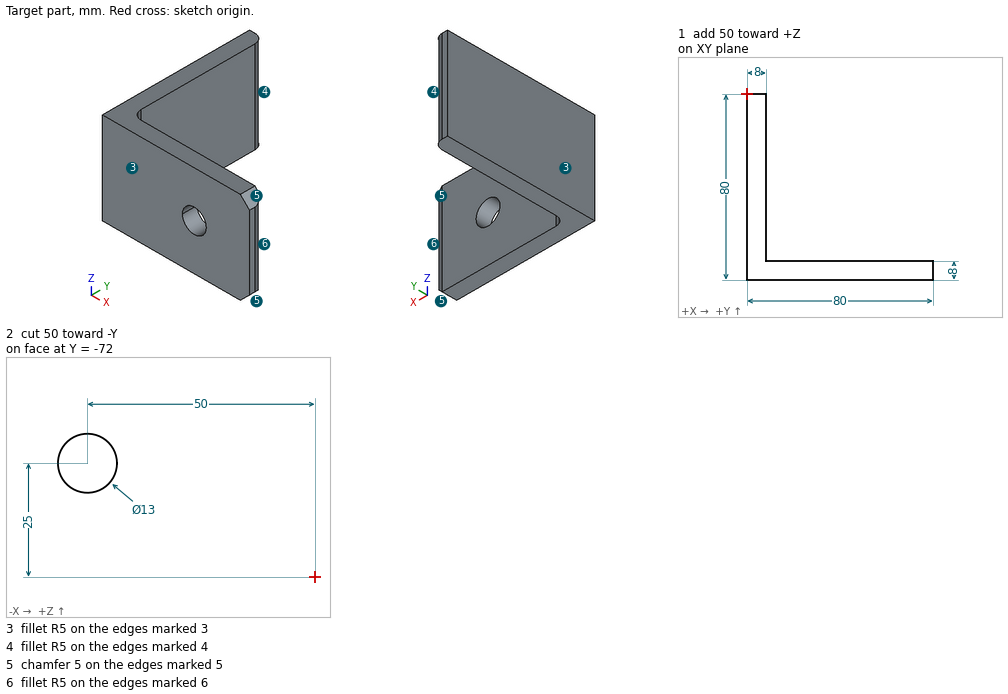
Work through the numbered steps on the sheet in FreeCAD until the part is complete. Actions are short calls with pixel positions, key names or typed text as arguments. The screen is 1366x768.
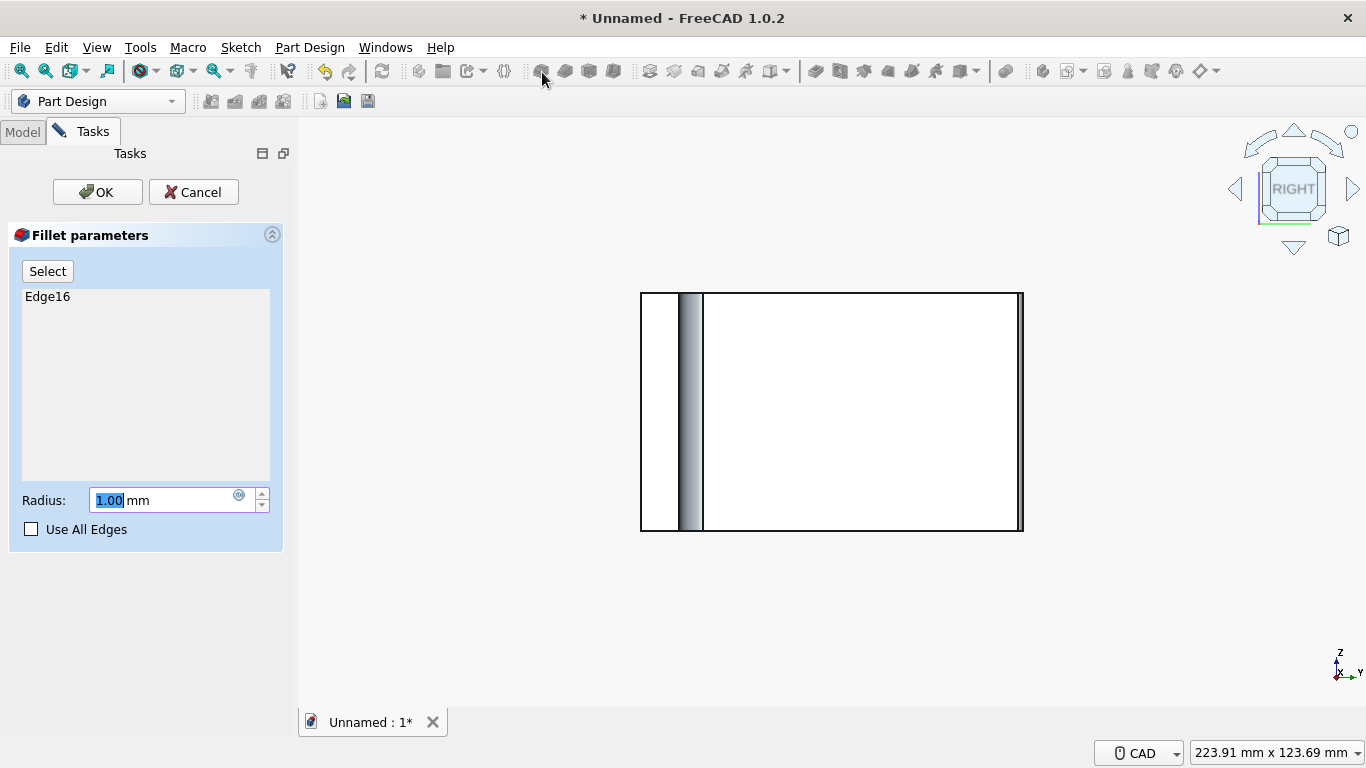
text(5)
key(Tab)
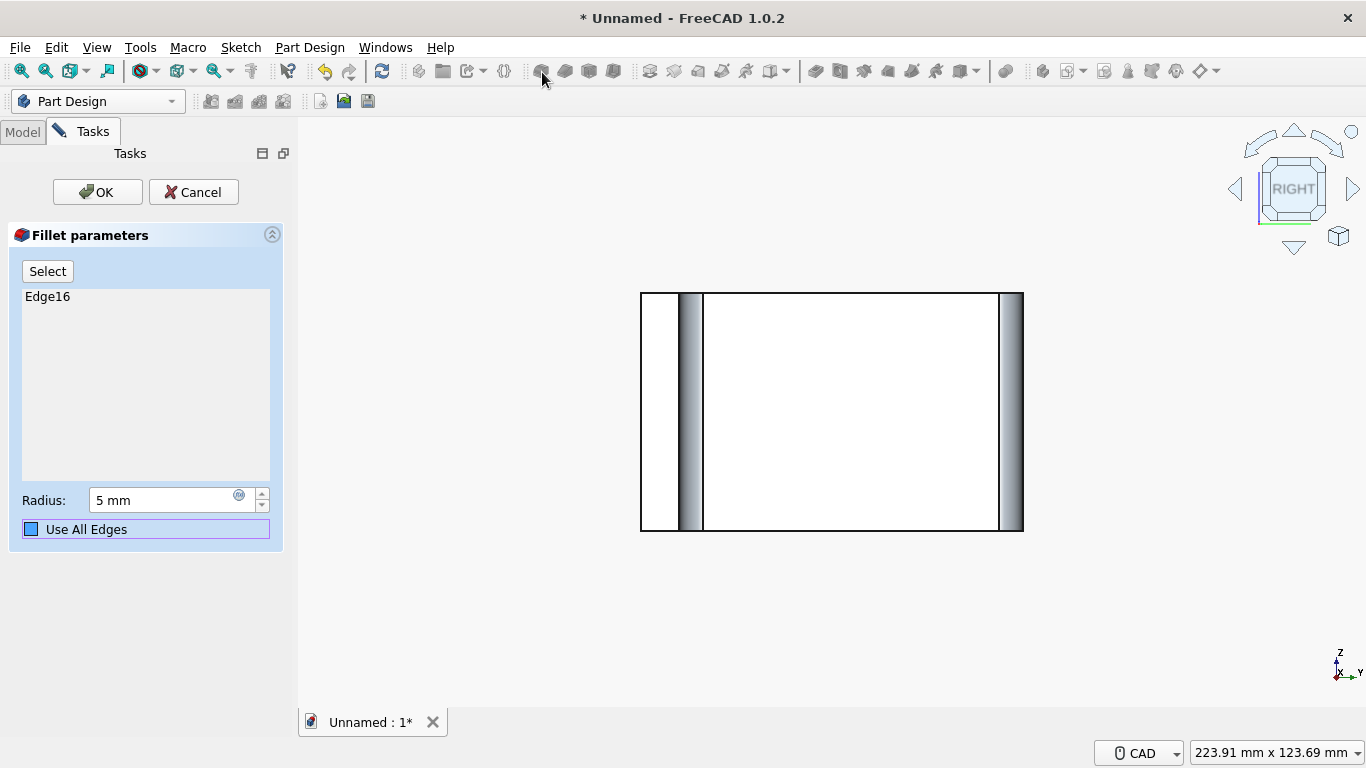
click(98, 192)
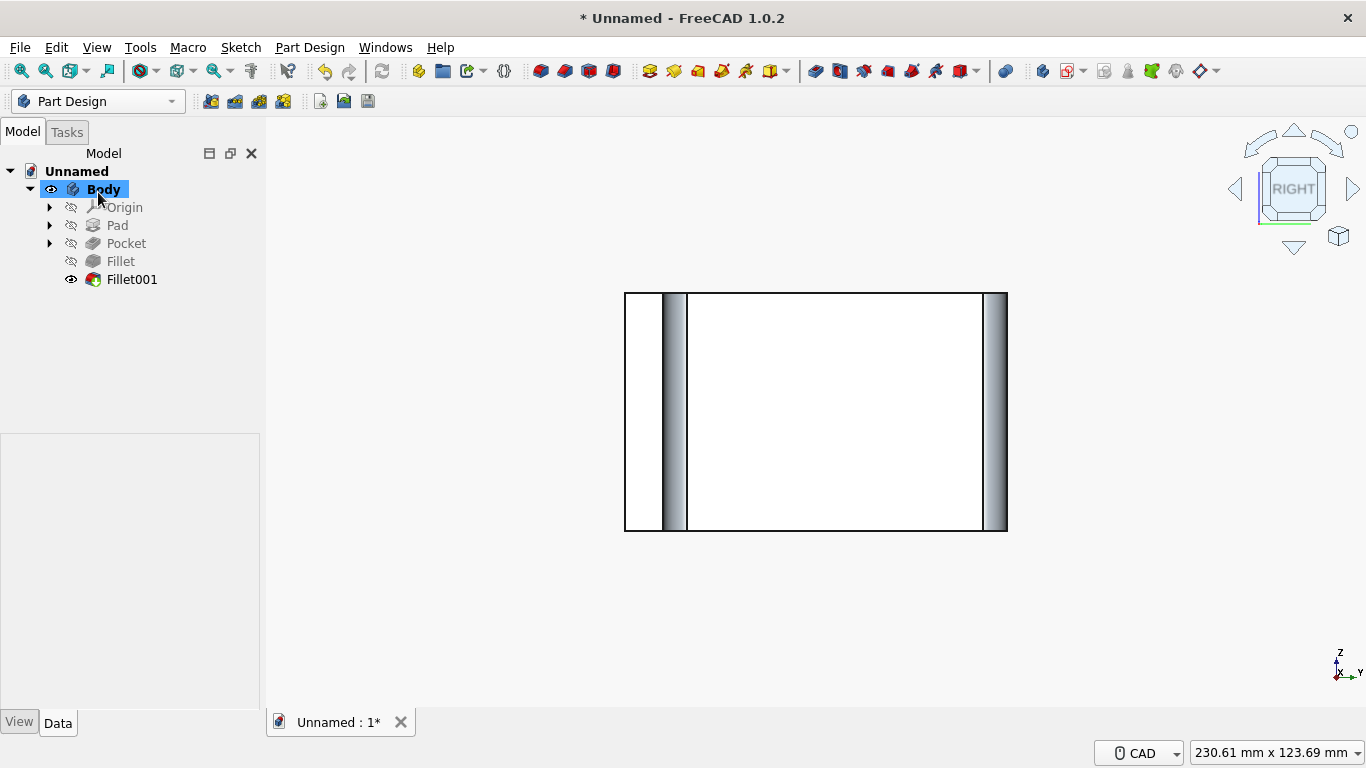
click(22, 72)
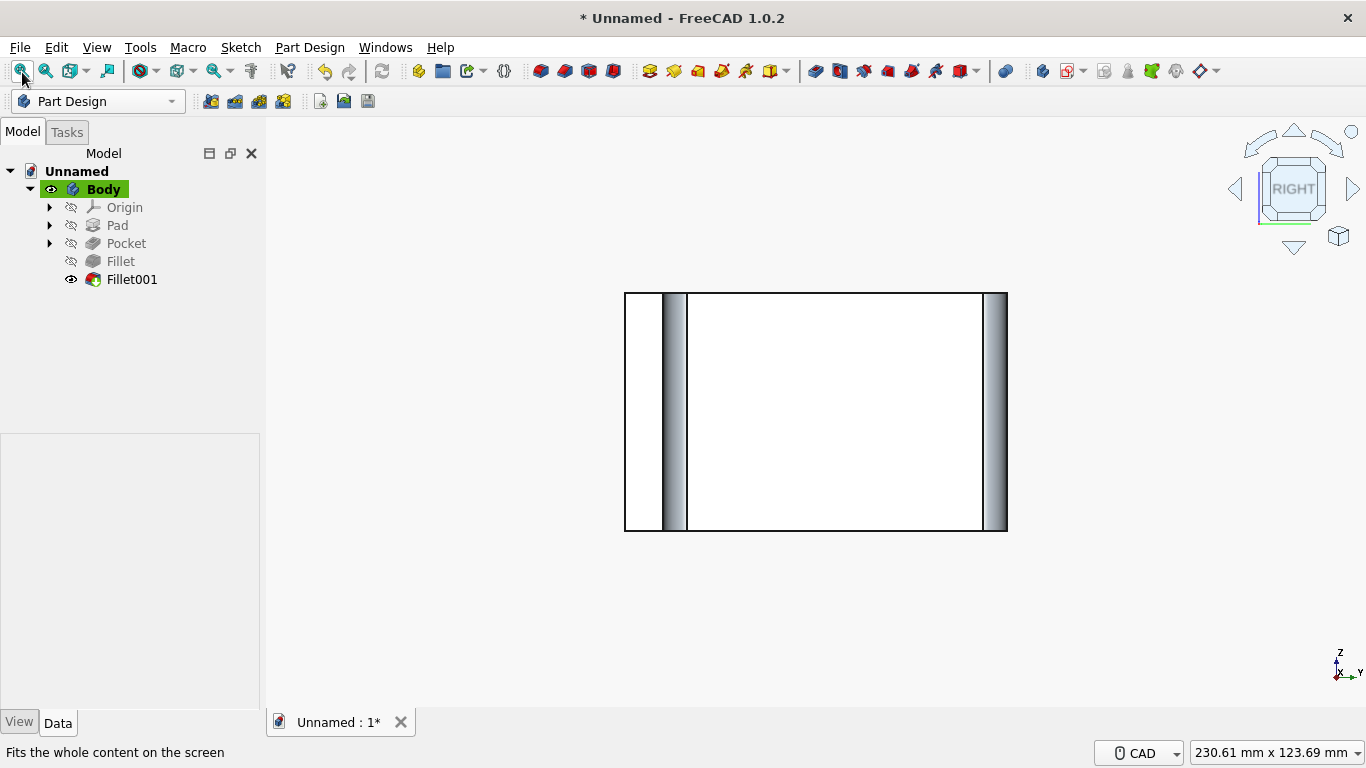
click(644, 530)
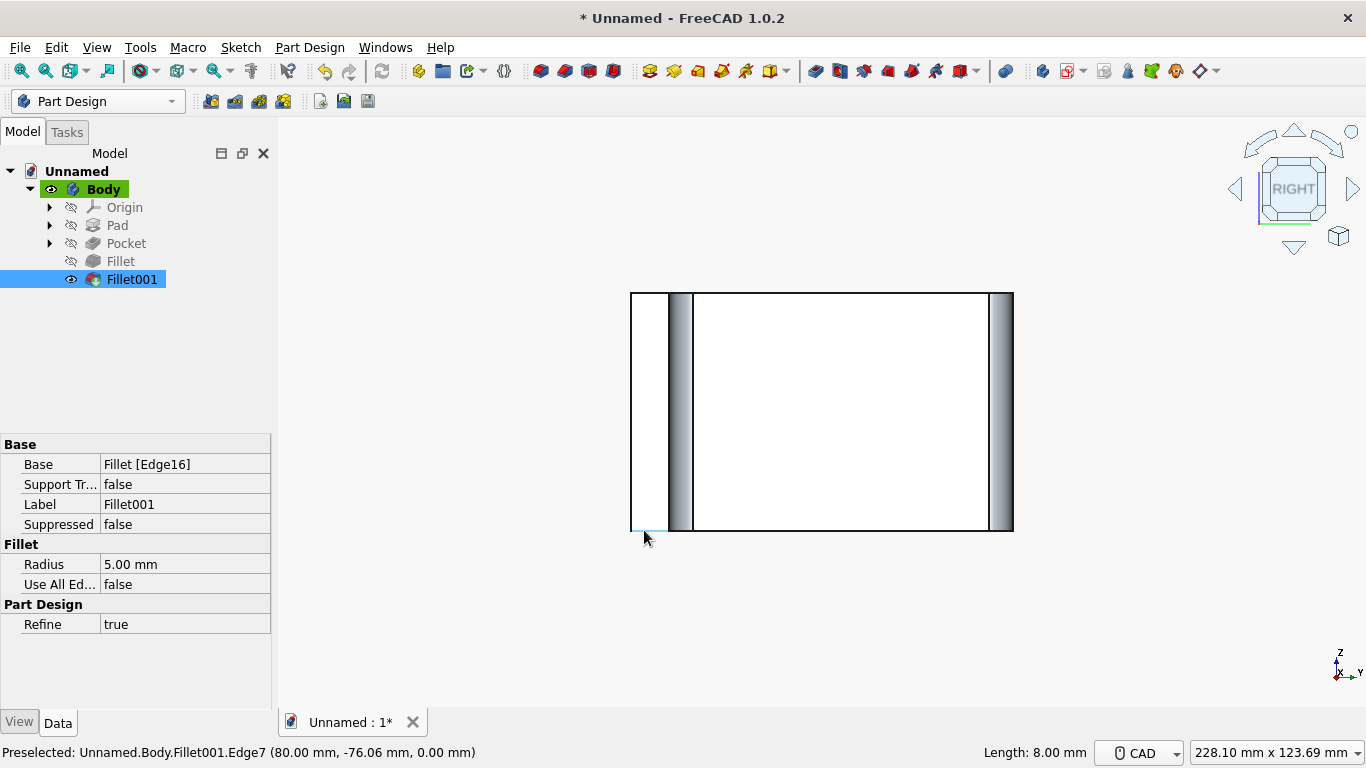
click(650, 292, ctrl)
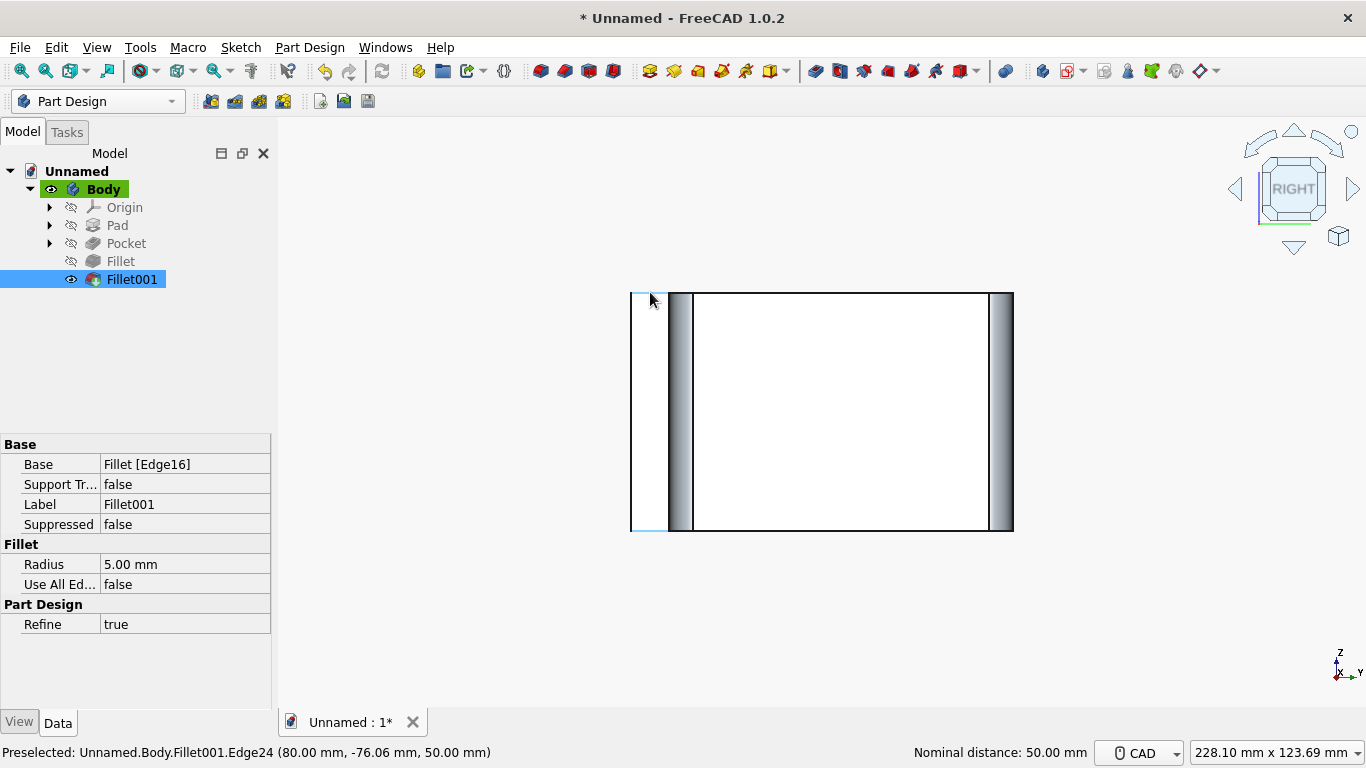
click(566, 72)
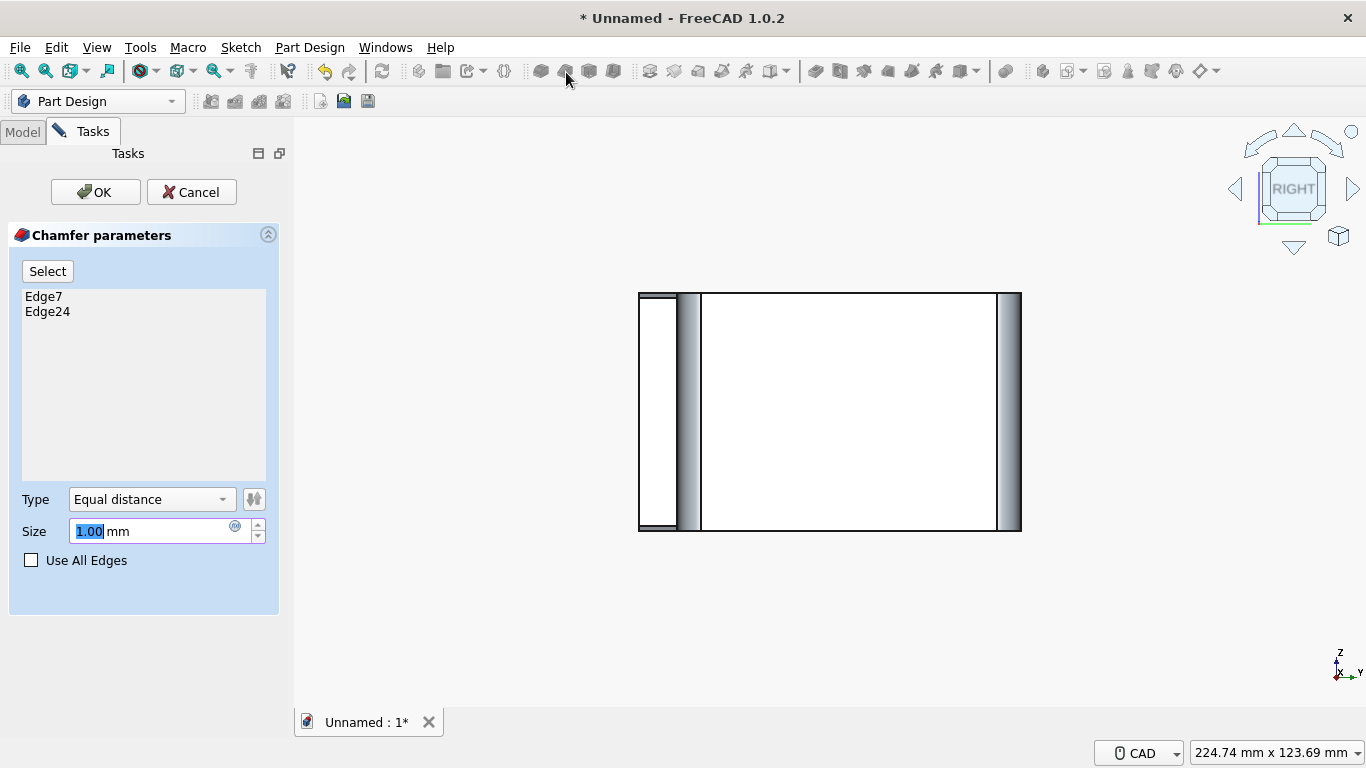
text(5)
key(Tab)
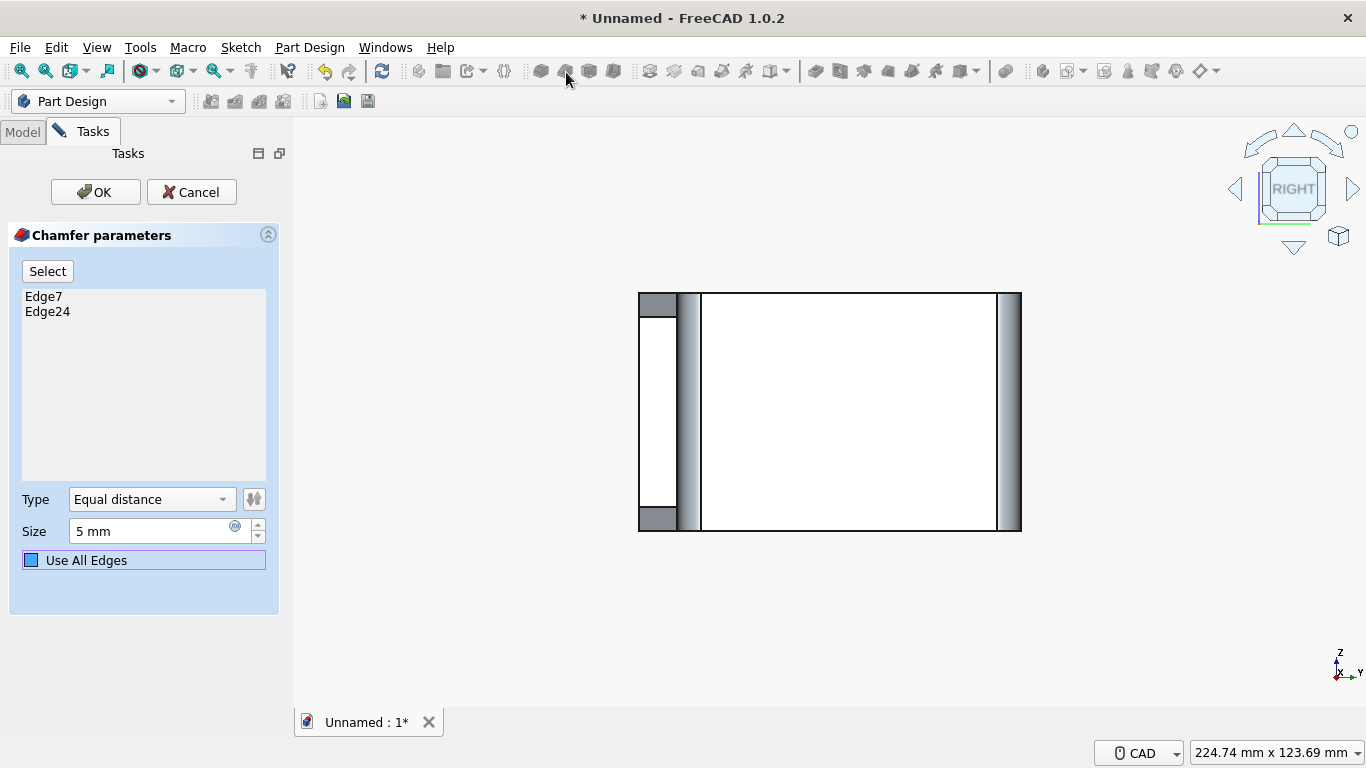
click(96, 192)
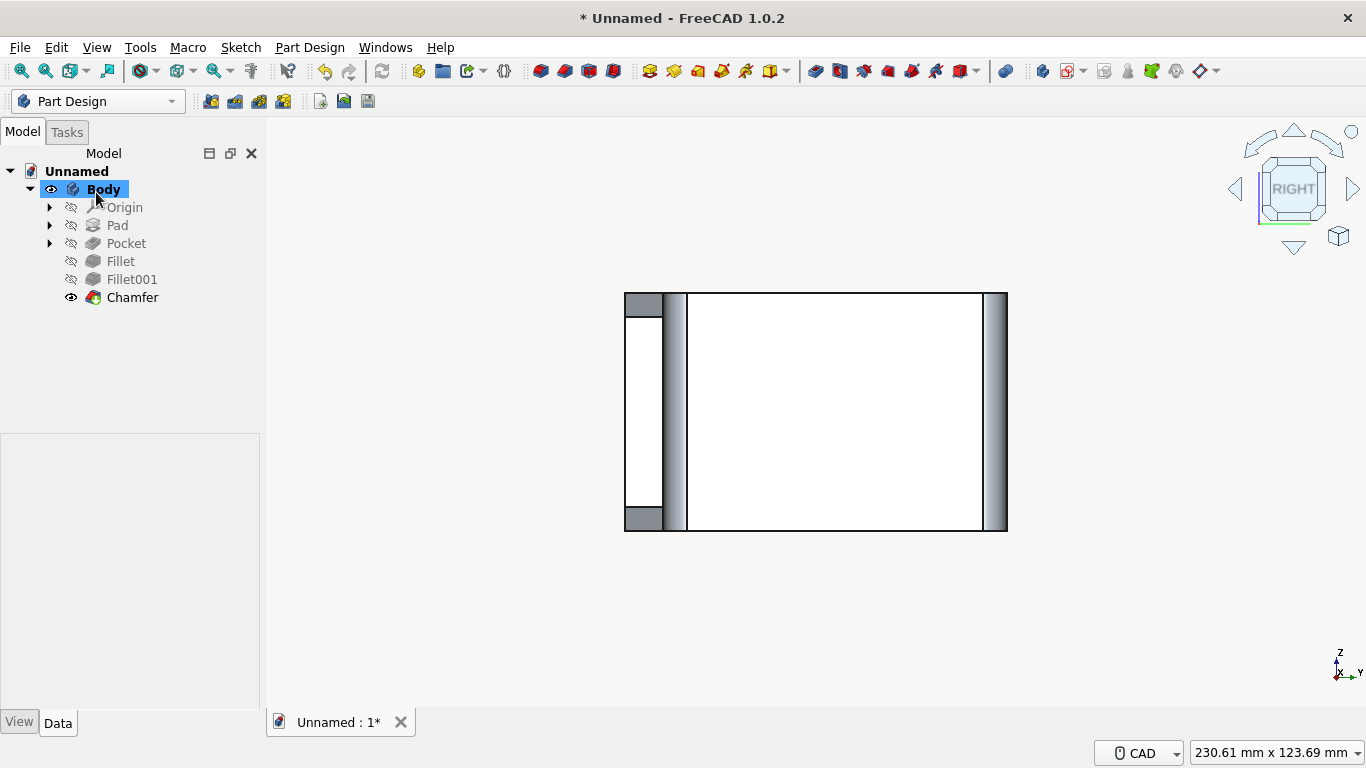
key(v)
key(f)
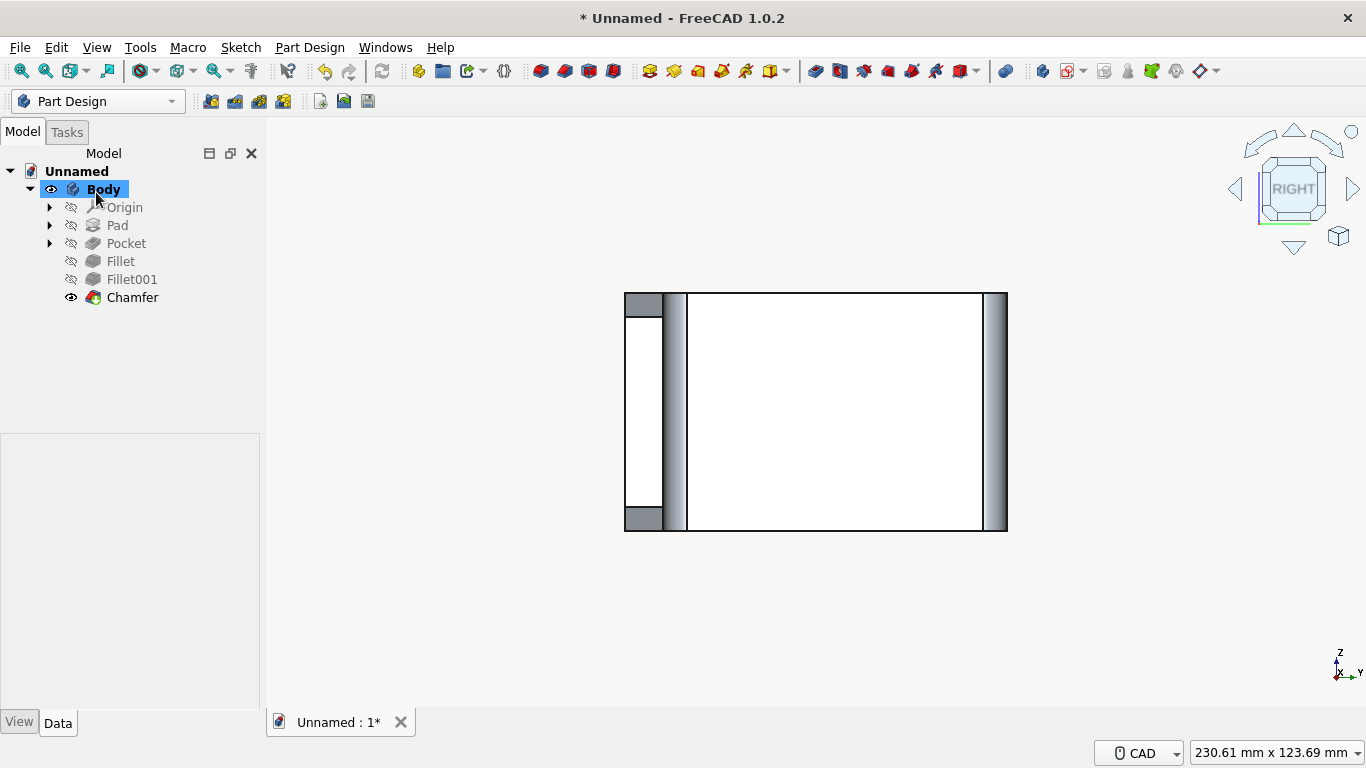
click(663, 411)